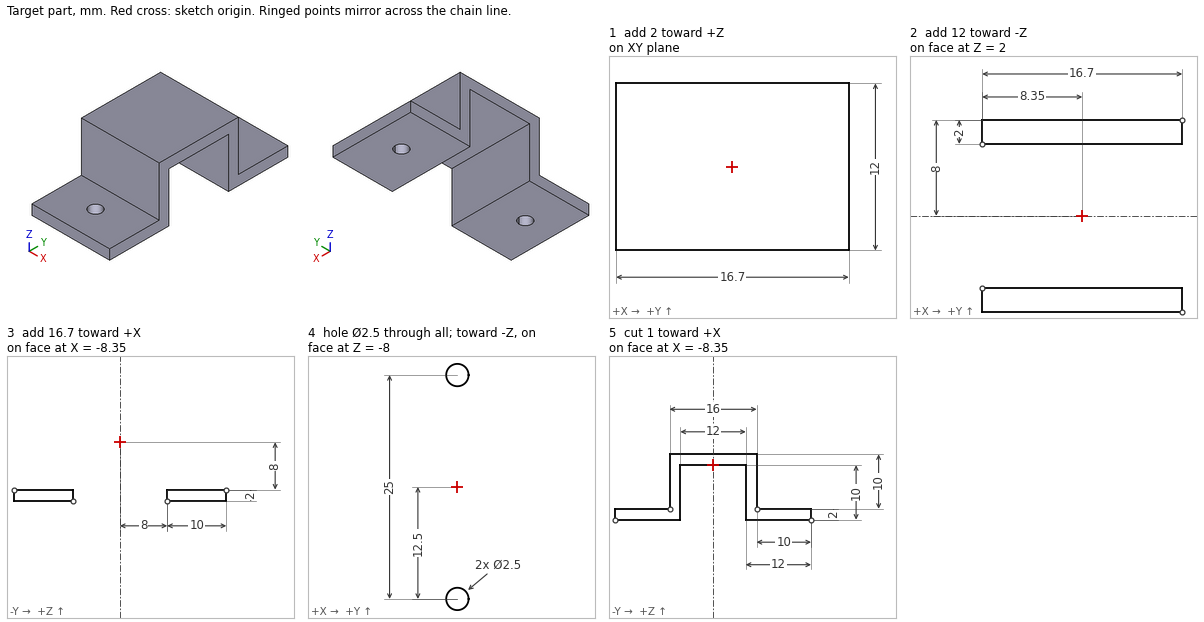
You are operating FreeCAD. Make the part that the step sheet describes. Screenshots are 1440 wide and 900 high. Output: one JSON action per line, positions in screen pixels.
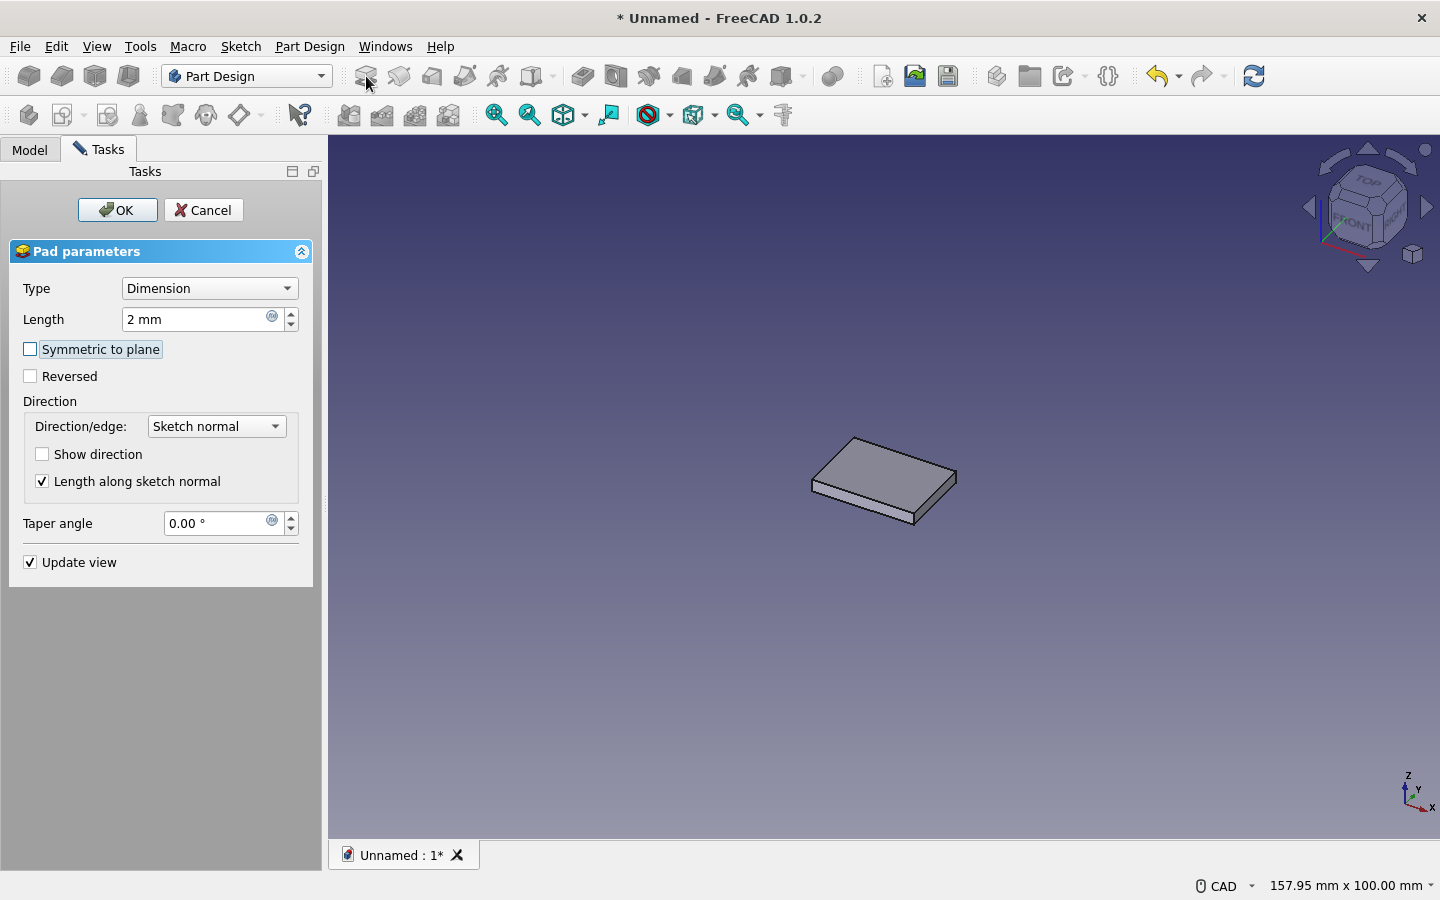
{"action": "left_click", "coordinate": [118, 210]}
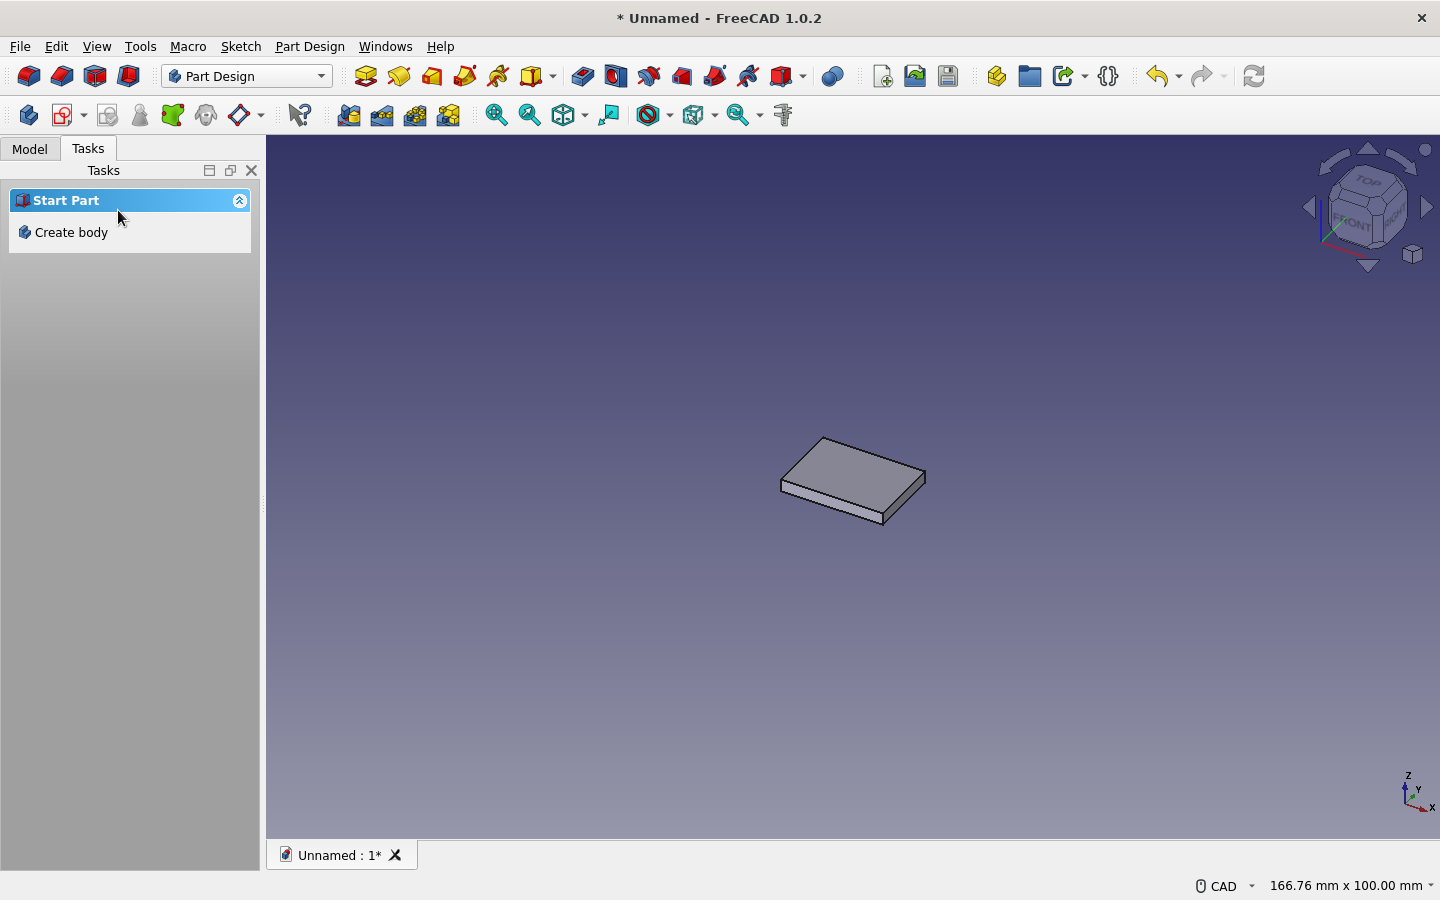
{"action": "left_click", "coordinate": [497, 116]}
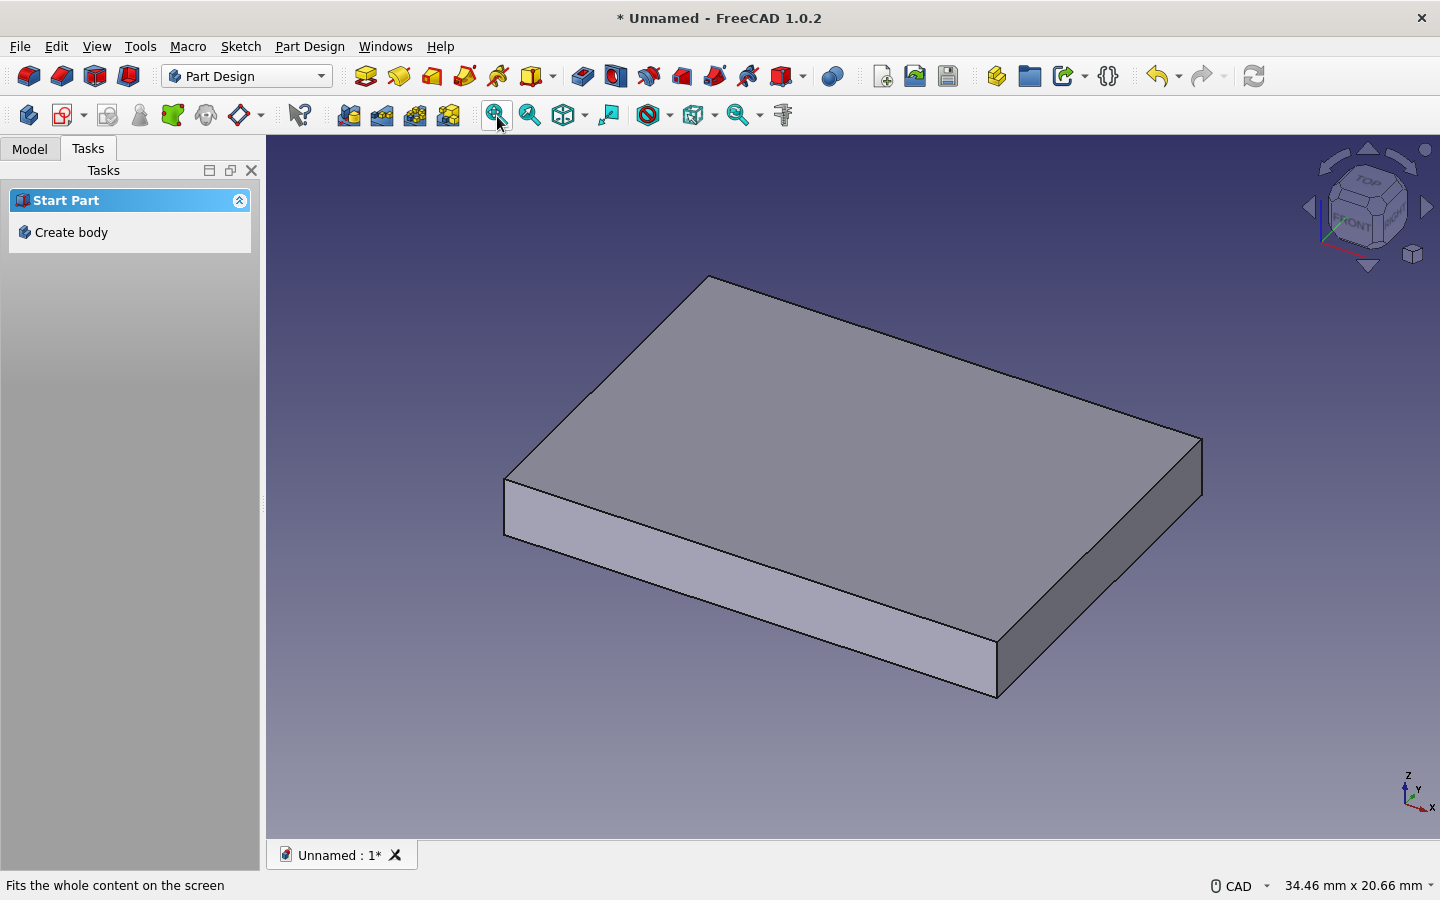
{"action": "left_click", "coordinate": [853, 458]}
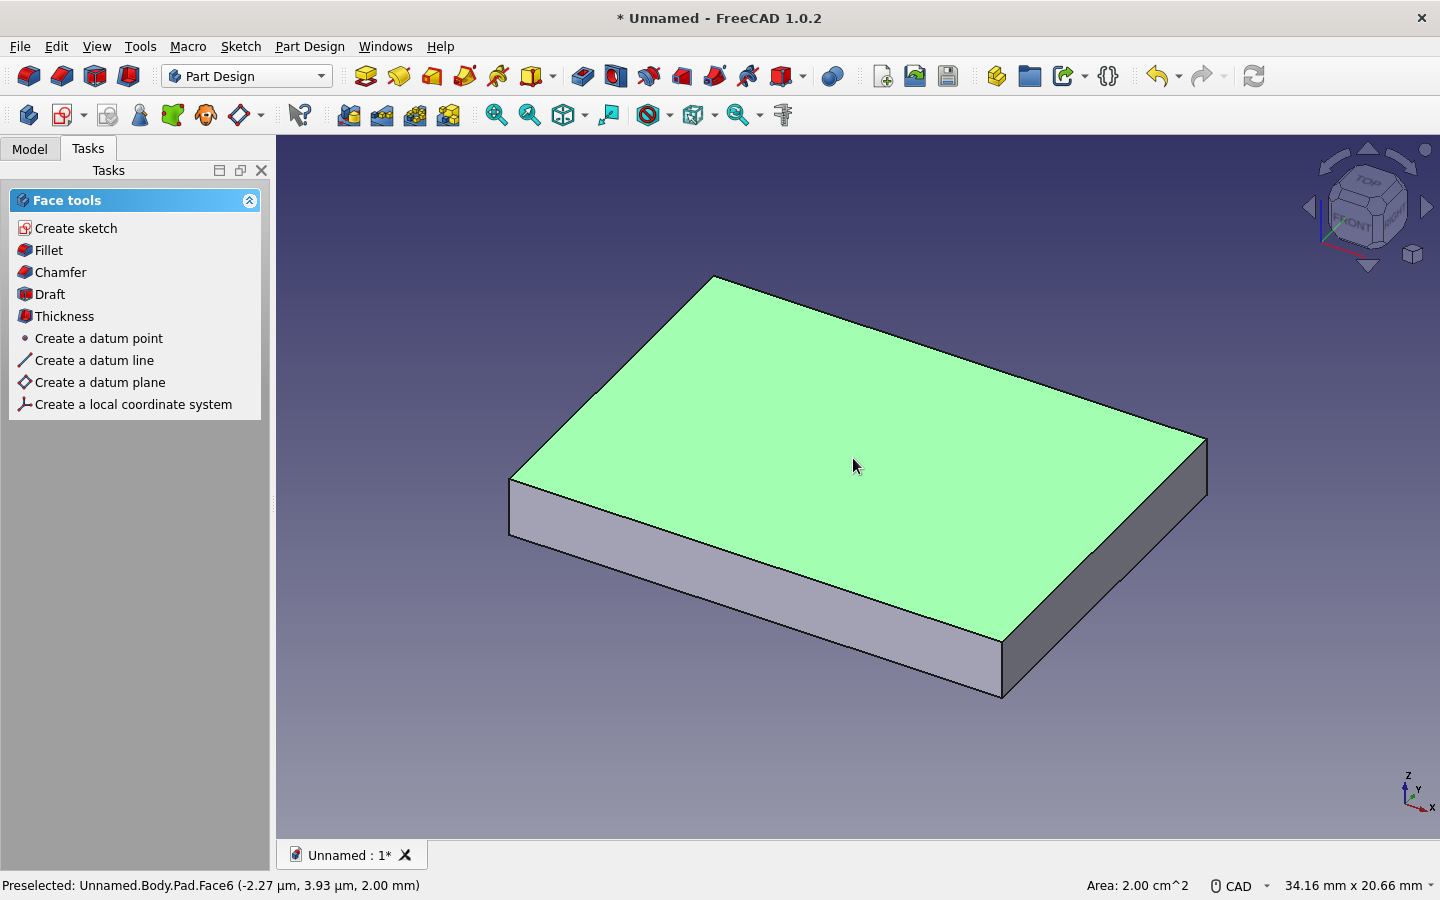
{"action": "left_click", "coordinate": [62, 116]}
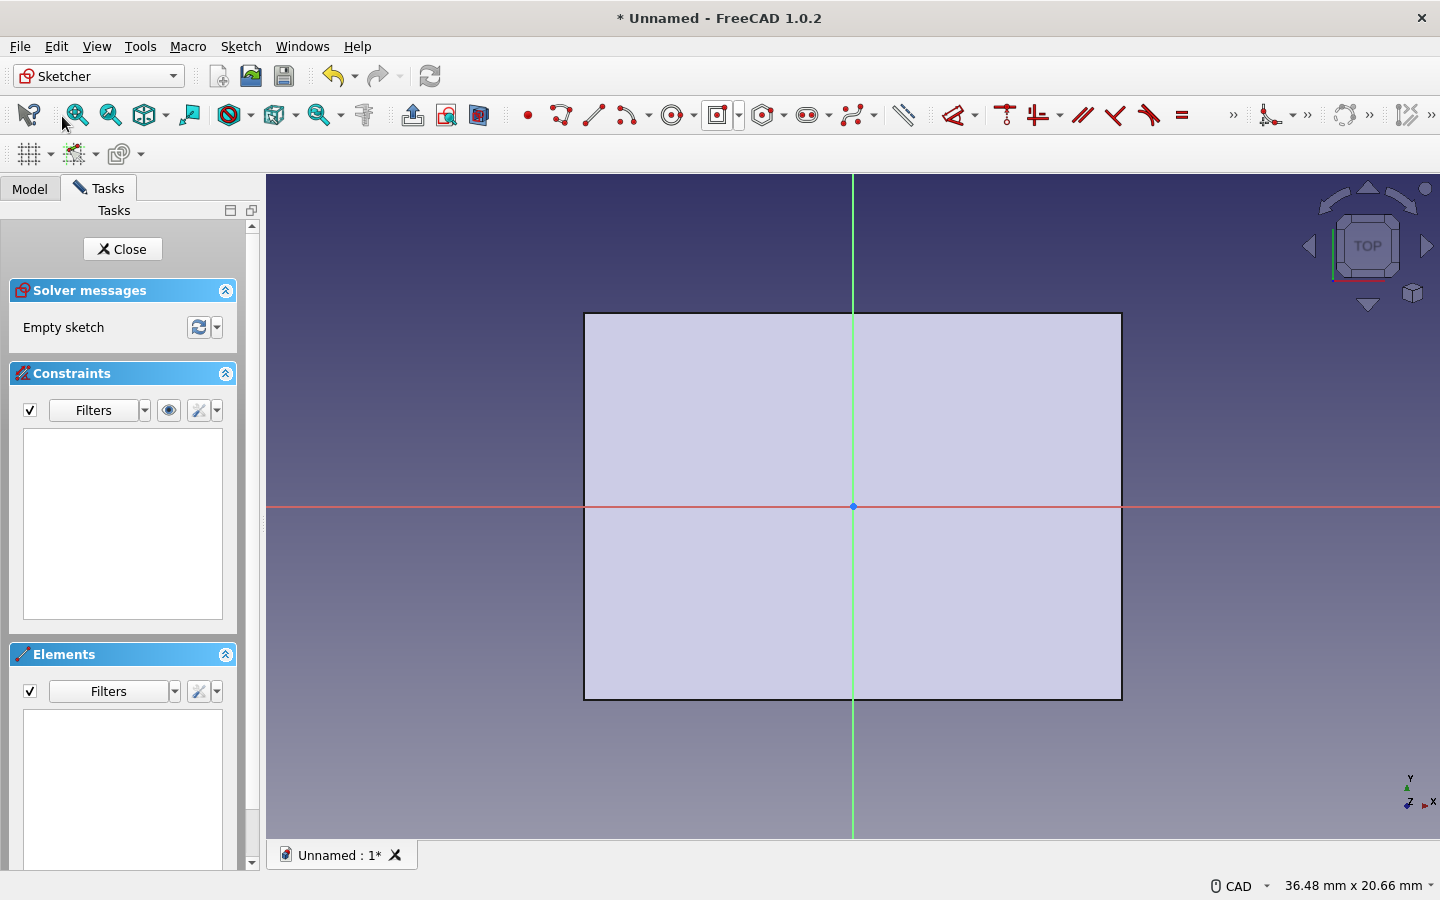
{"action": "key", "text": "g r"}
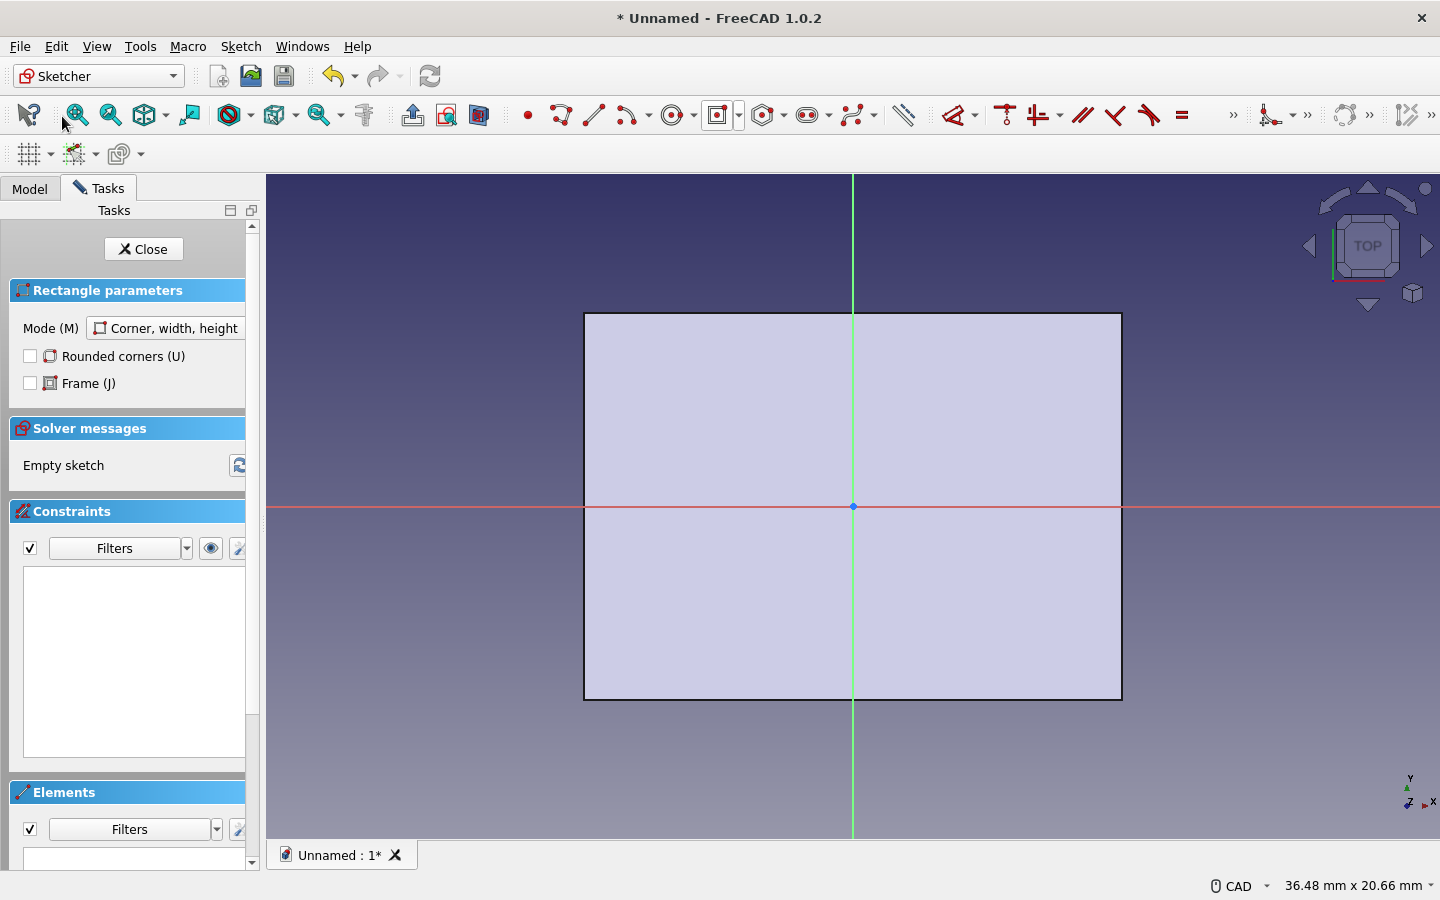
{"action": "left_click", "coordinate": [584, 249]}
{"action": "left_click", "coordinate": [1122, 313]}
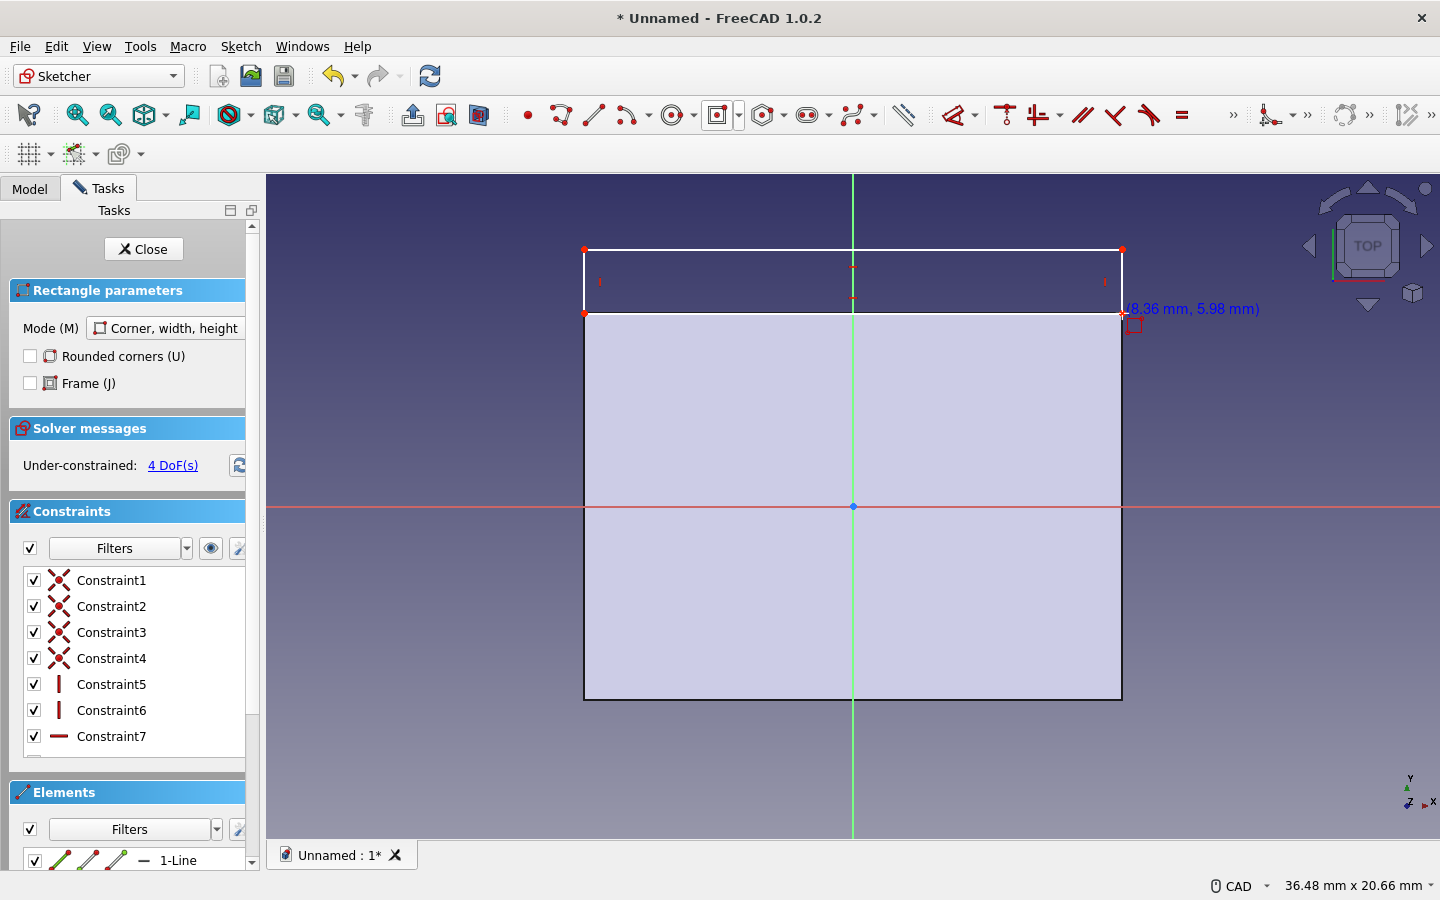
{"action": "left_click", "coordinate": [584, 700]}
{"action": "left_click", "coordinate": [1122, 764]}
{"action": "key", "text": "Escape"}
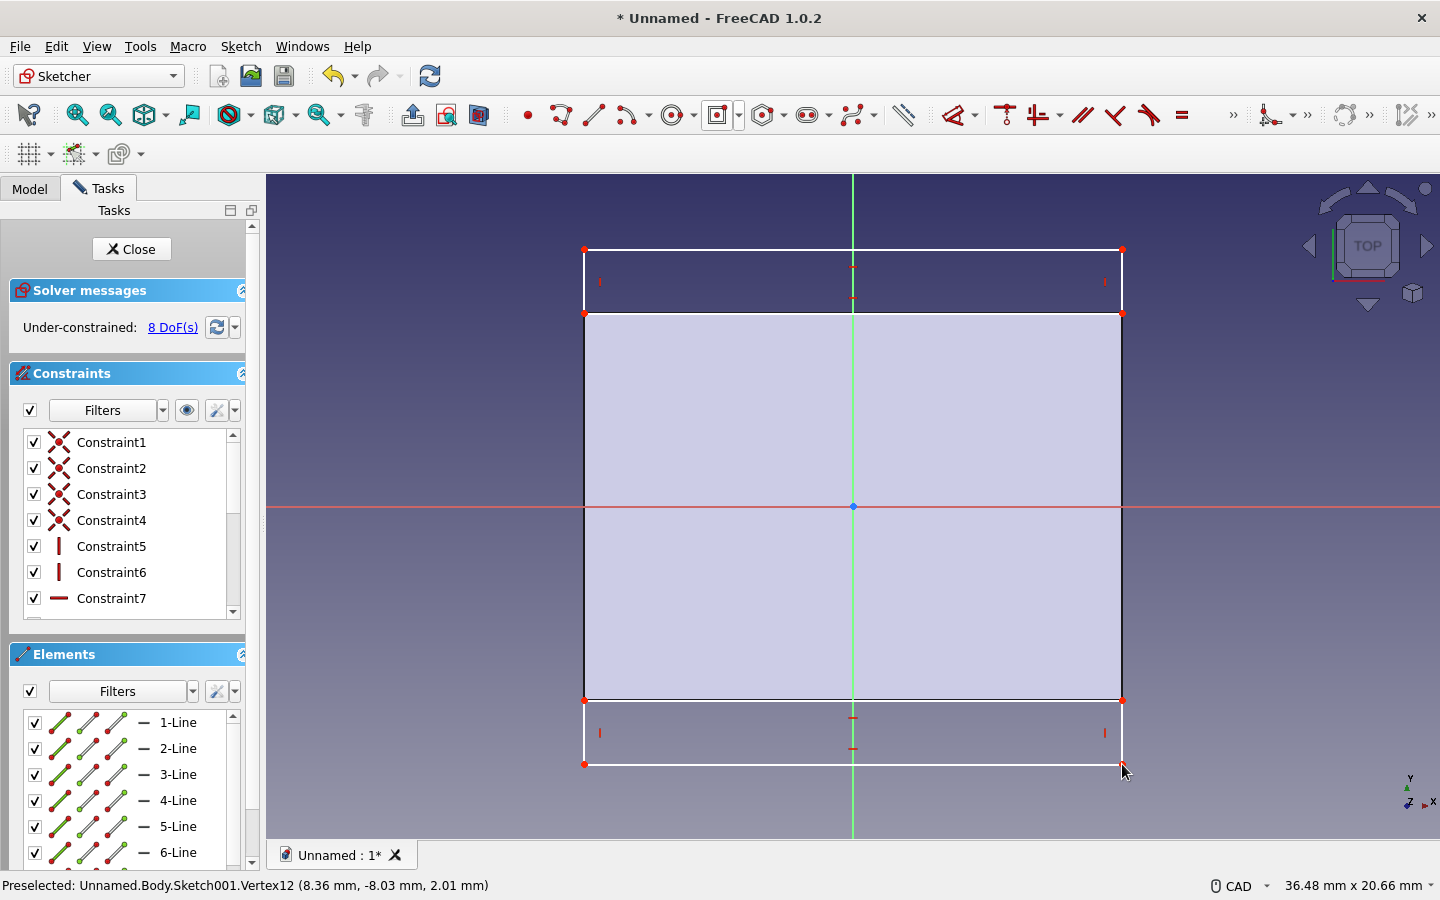
{"action": "left_click", "coordinate": [584, 314]}